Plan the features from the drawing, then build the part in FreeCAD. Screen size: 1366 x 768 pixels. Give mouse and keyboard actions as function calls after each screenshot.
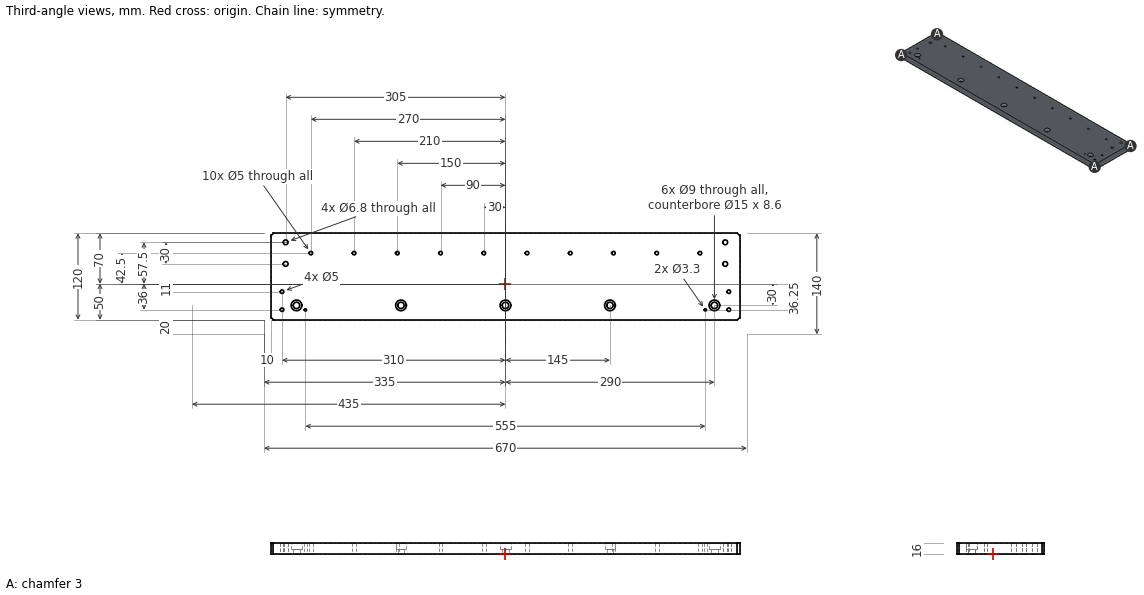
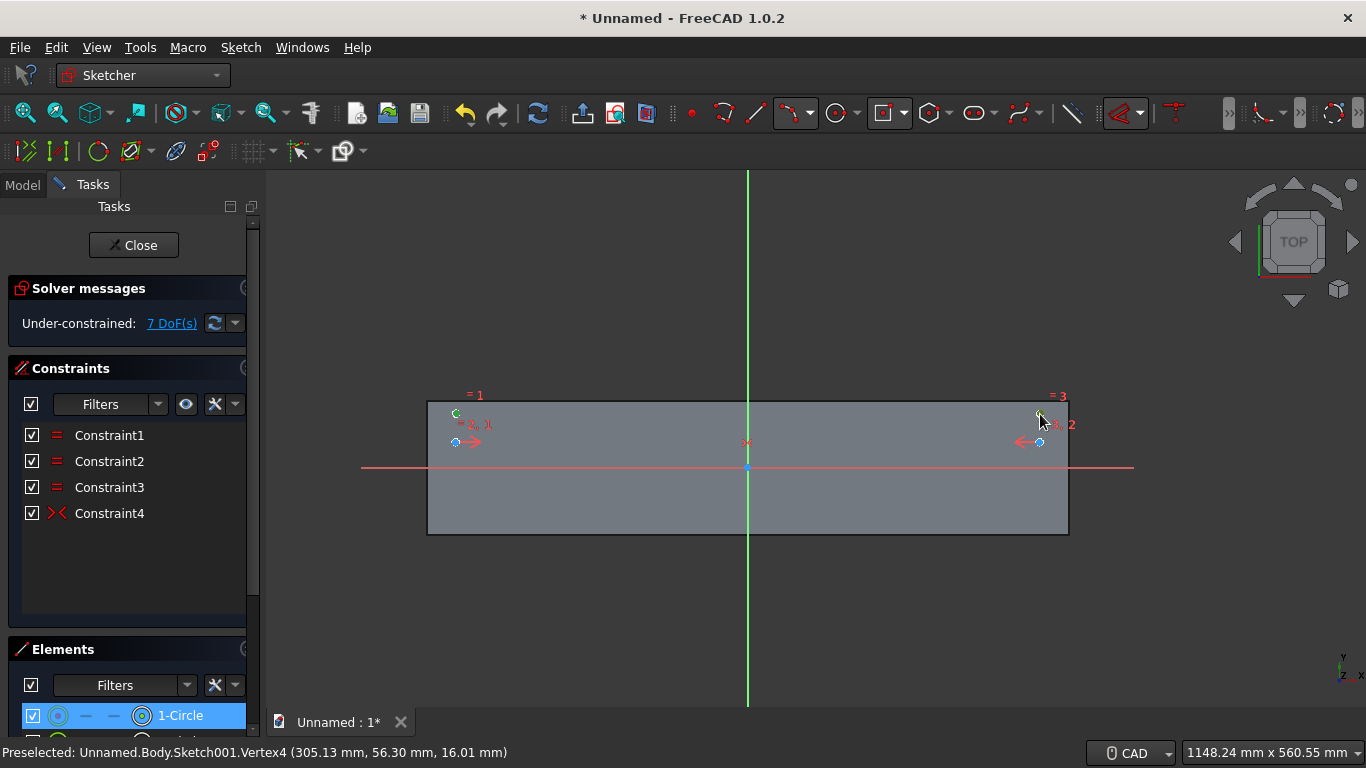
click(748, 645)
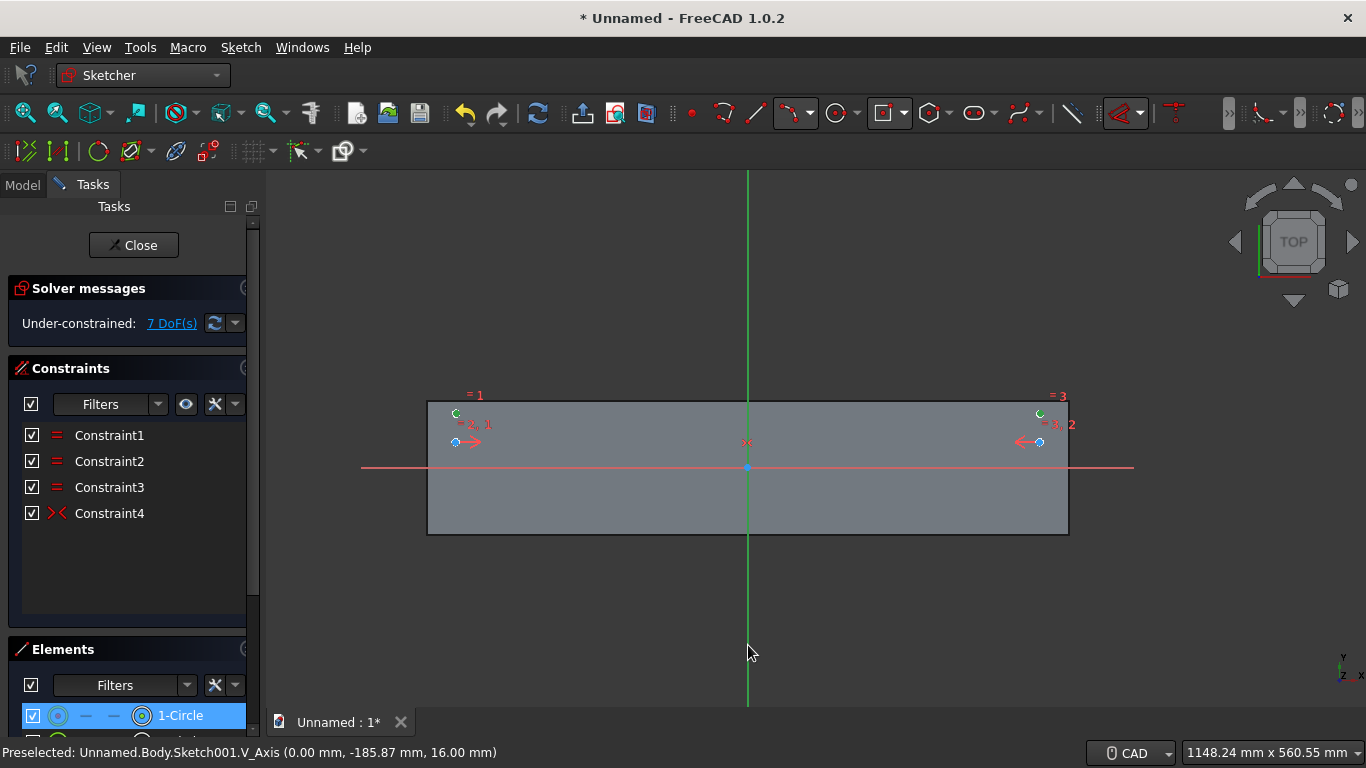
key(s)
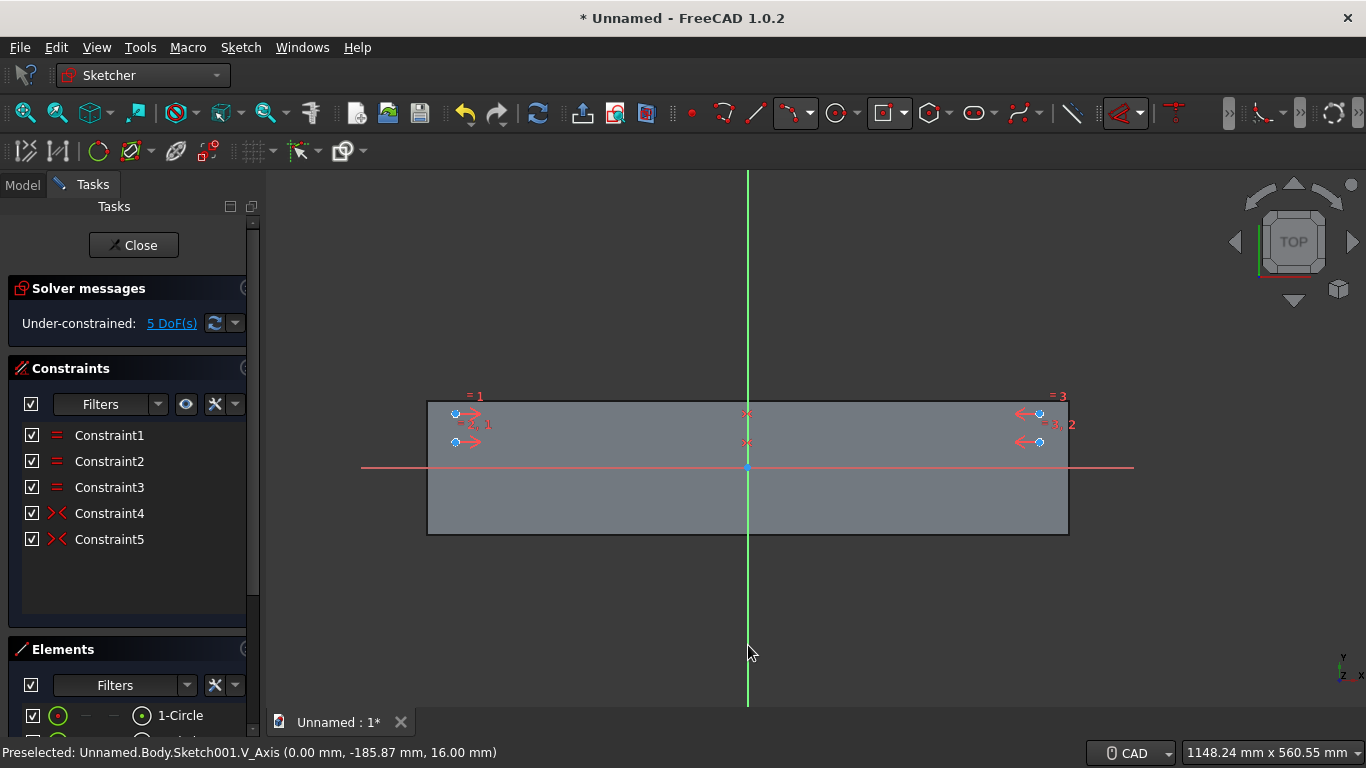
scroll(458, 416, up, 10)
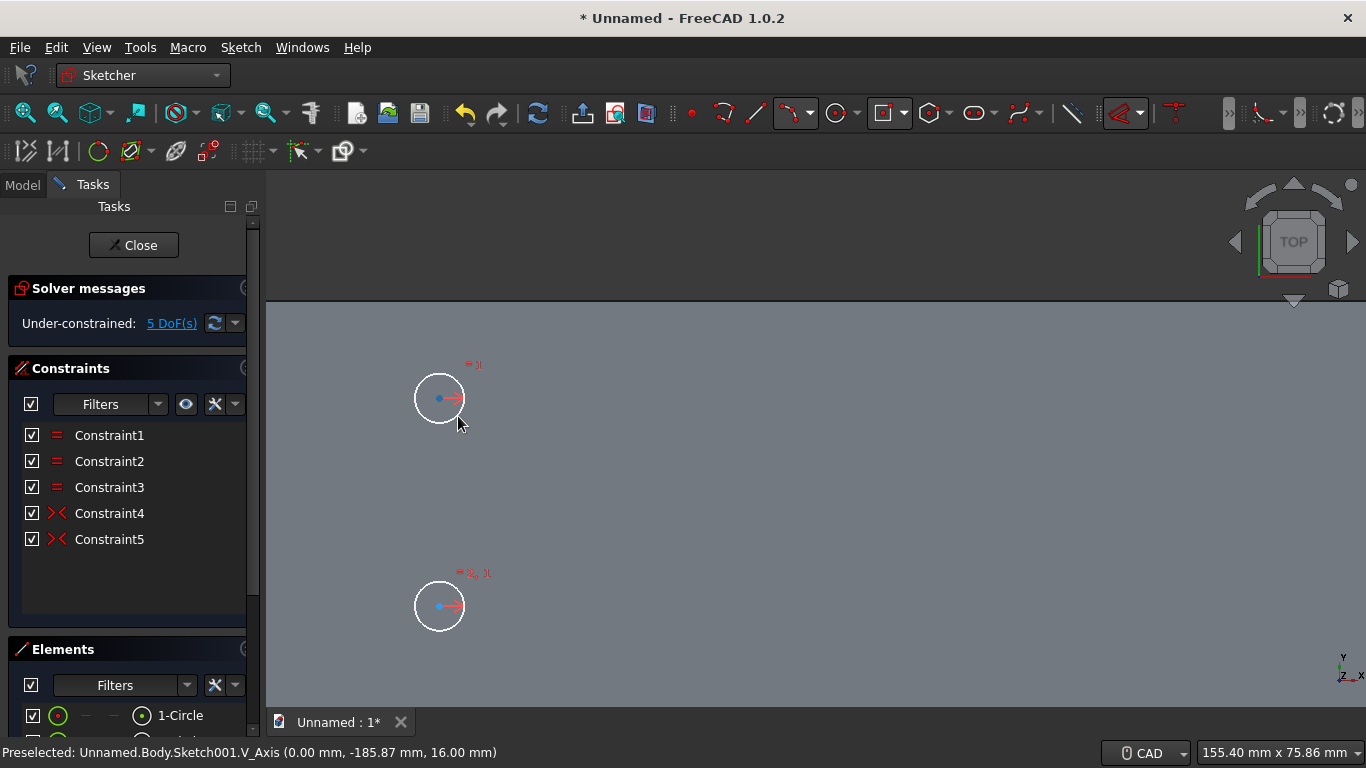
click(457, 416)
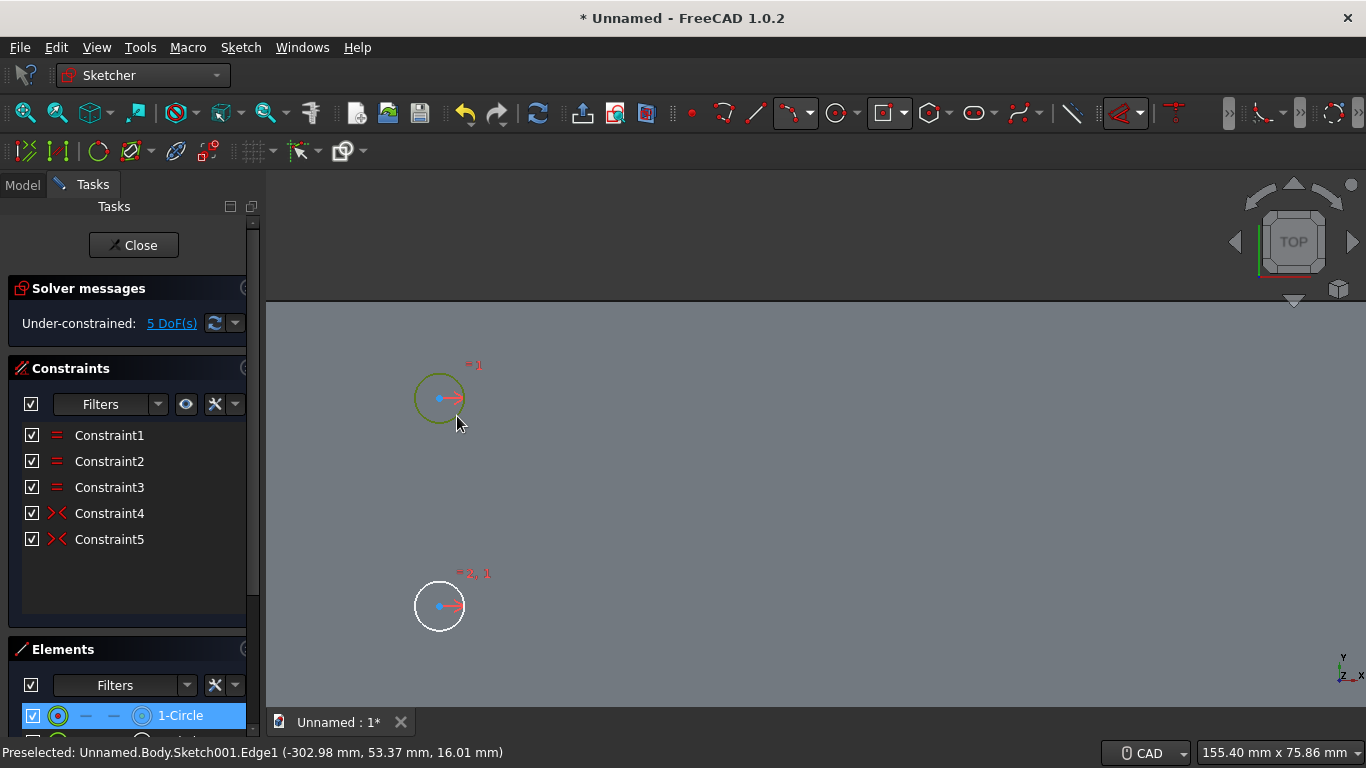
click(1142, 114)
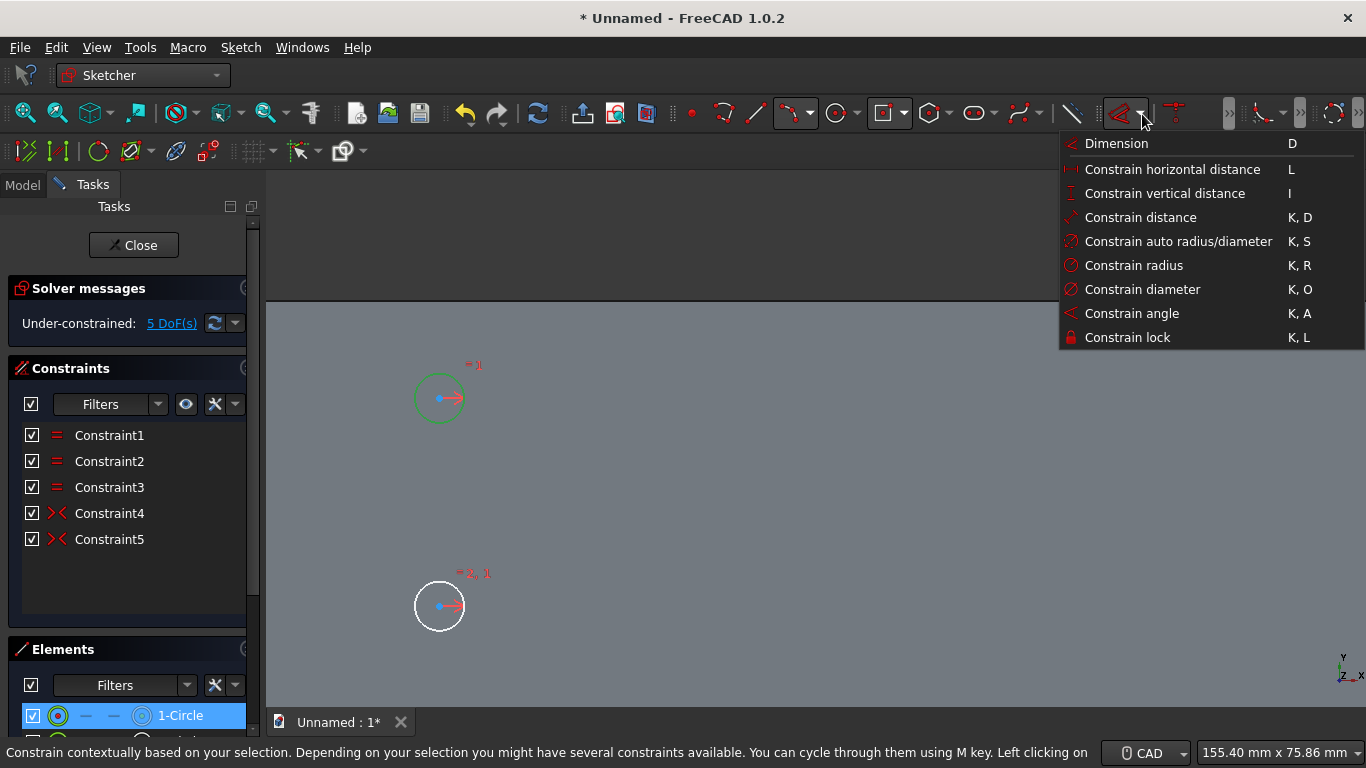
click(1212, 289)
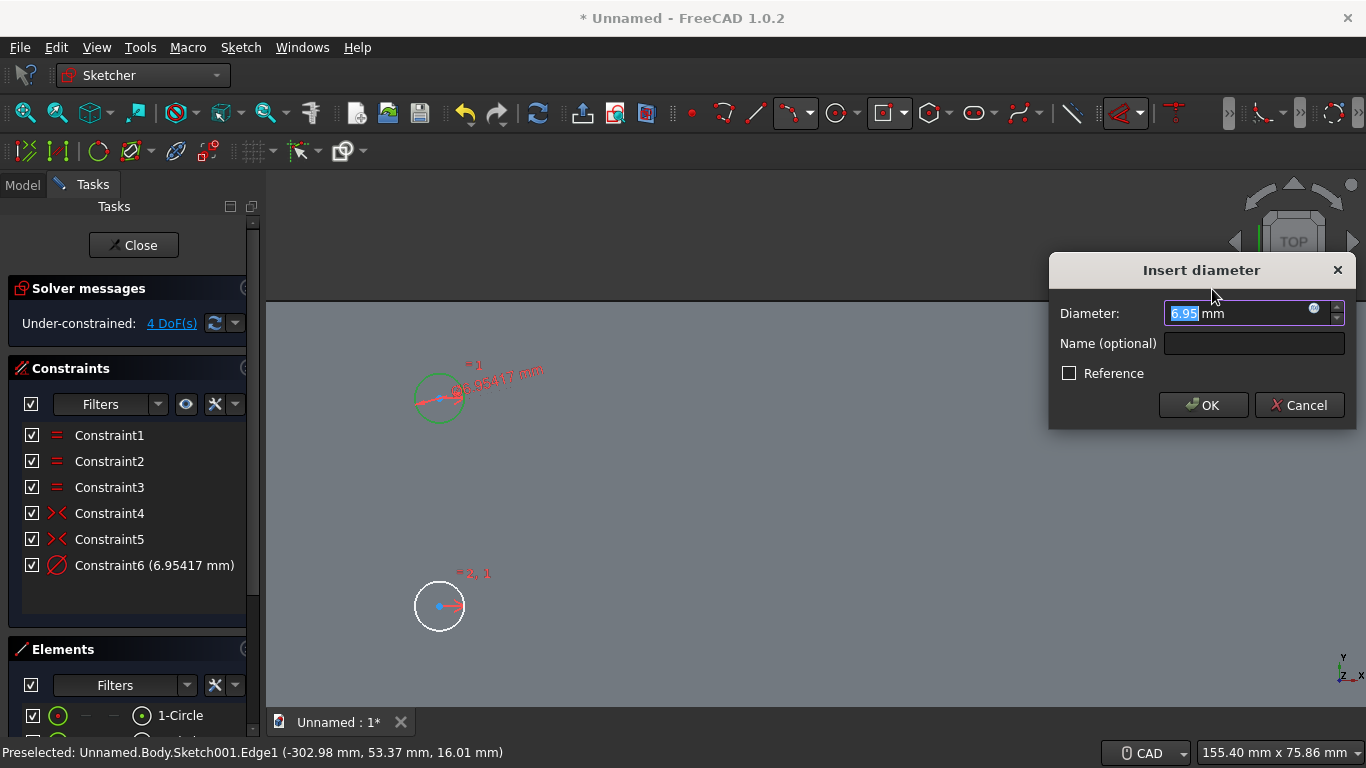
text(6.8)
key(Return)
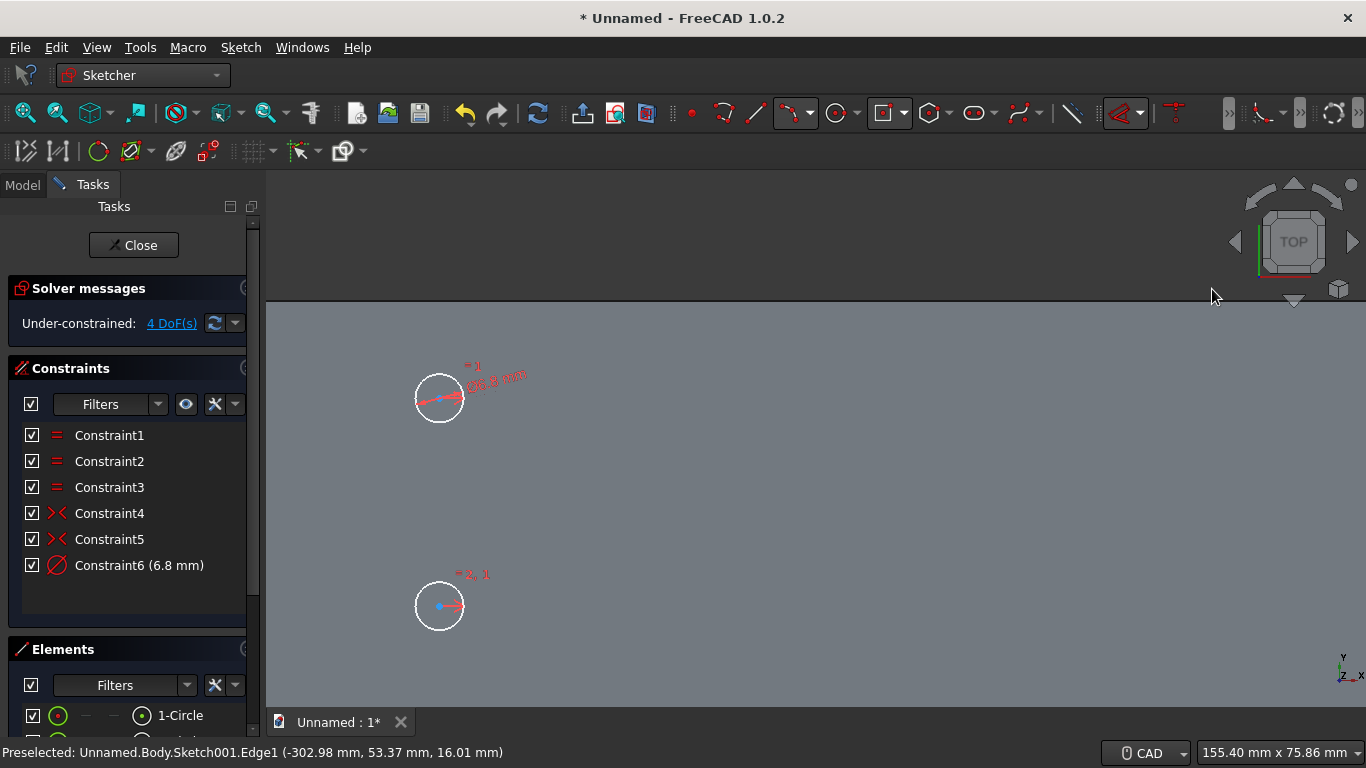
scroll(458, 416, down, 10)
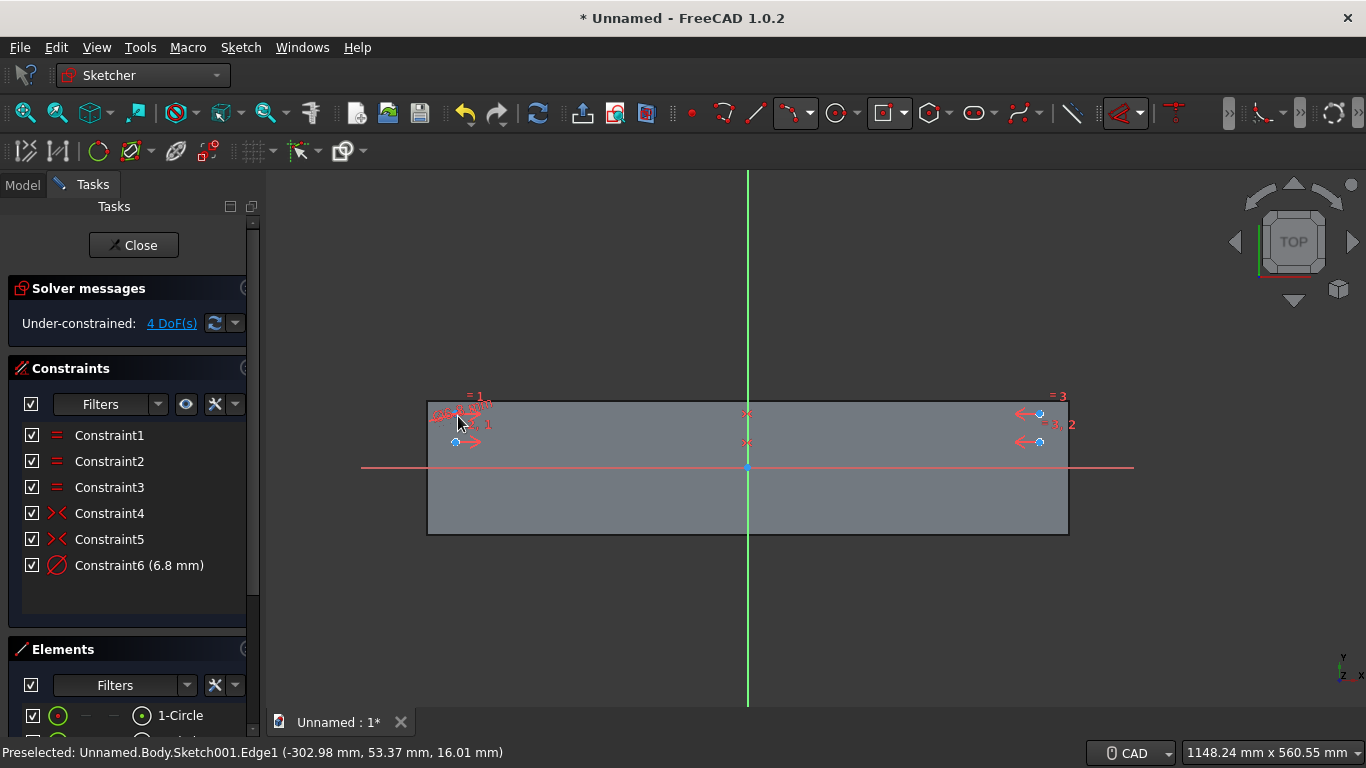
click(456, 414)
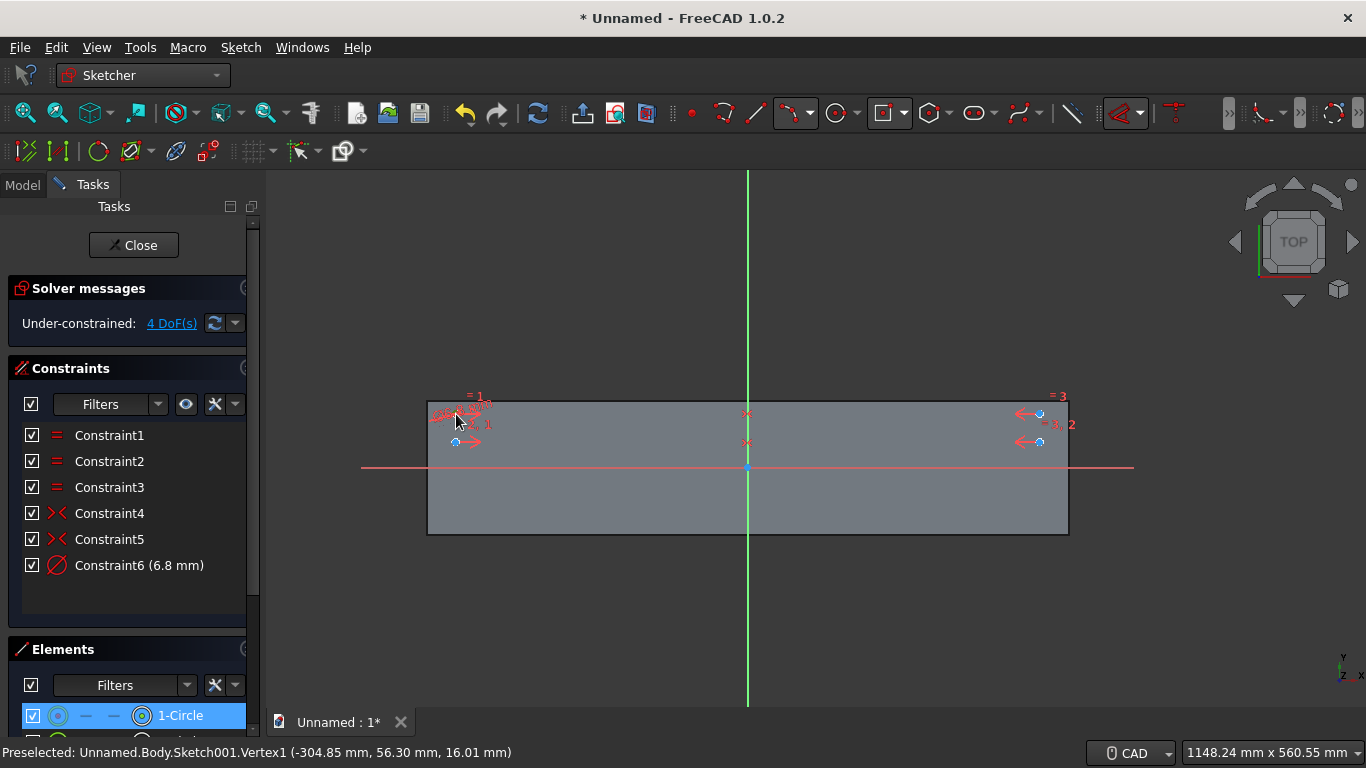
click(1142, 114)